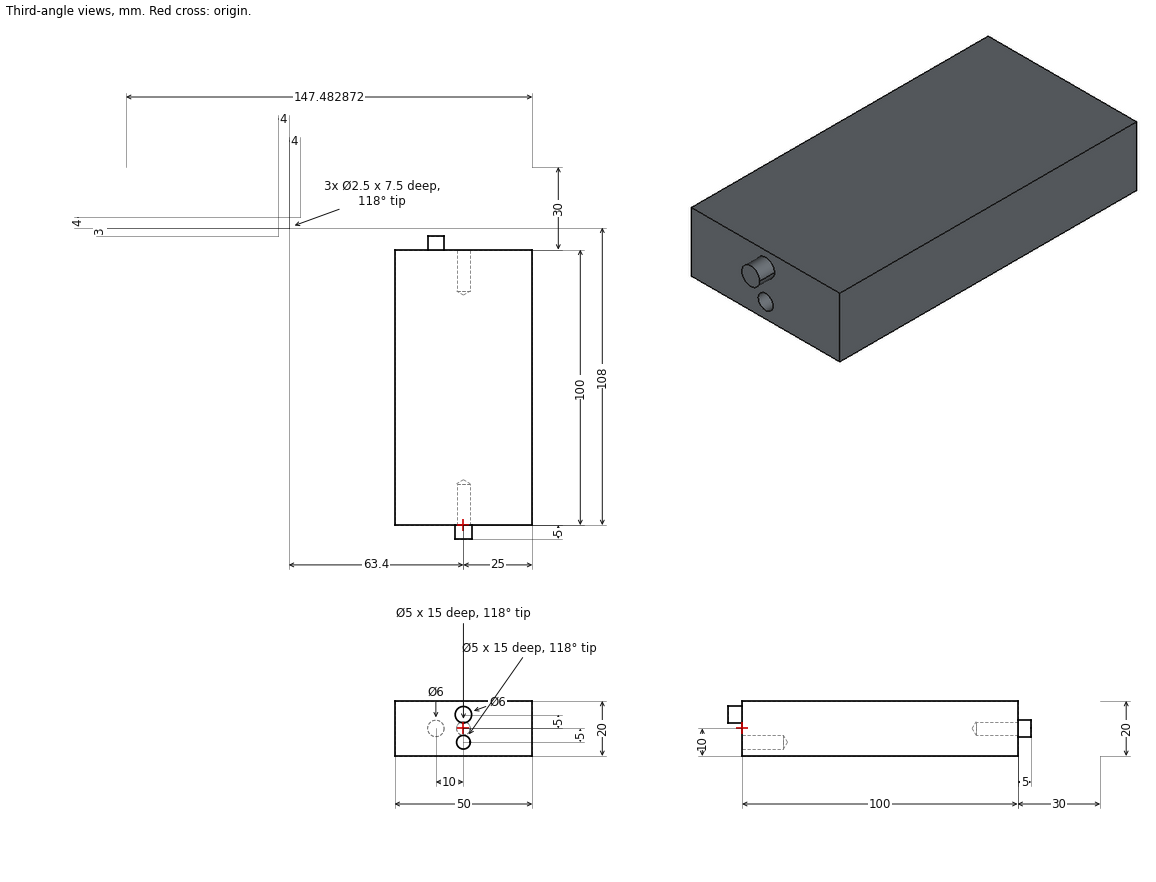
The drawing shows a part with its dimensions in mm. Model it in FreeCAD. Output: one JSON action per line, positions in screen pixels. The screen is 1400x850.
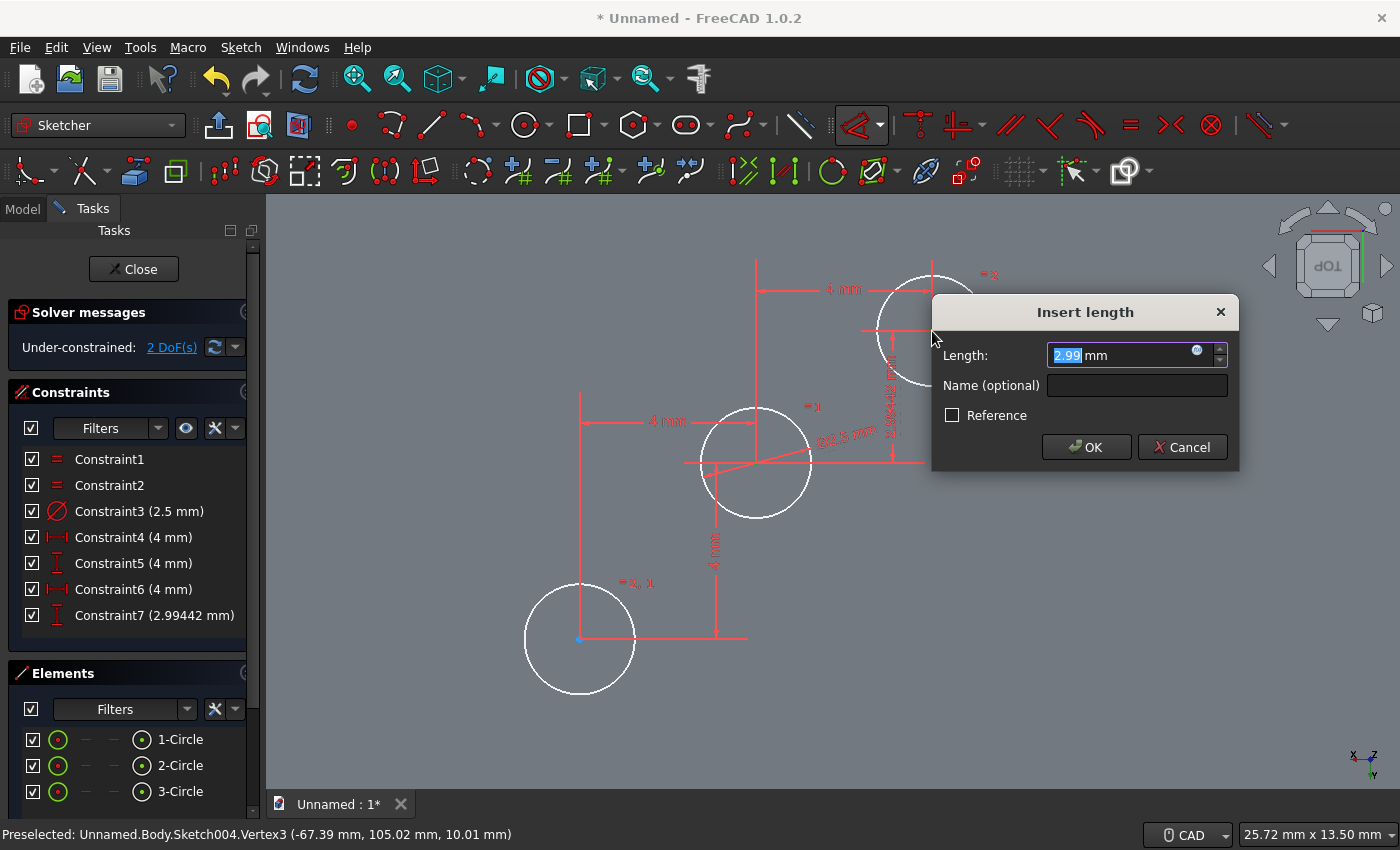
{"action": "type", "text": "3"}
{"action": "key", "text": "Return"}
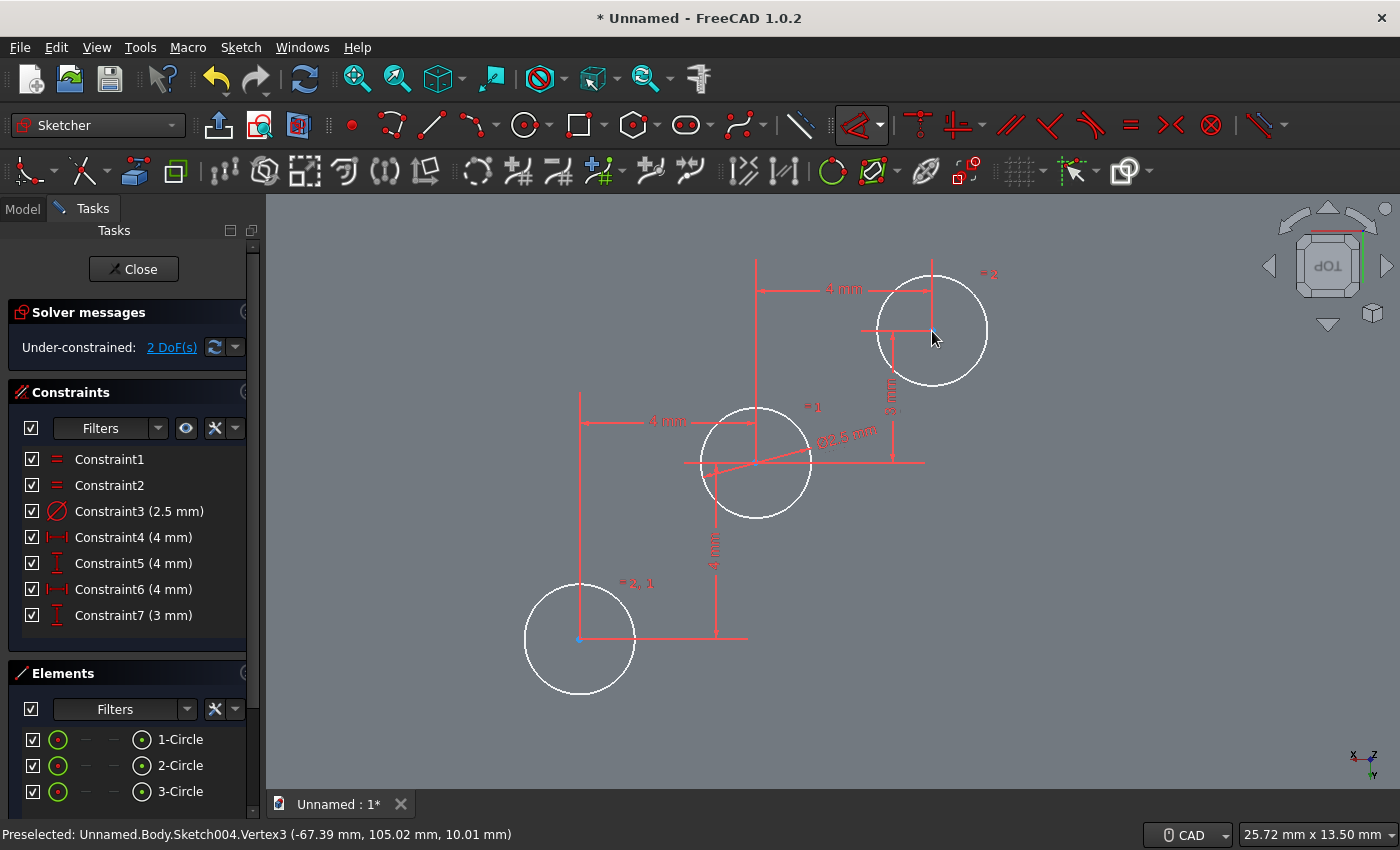
{"action": "left_click", "coordinate": [756, 463]}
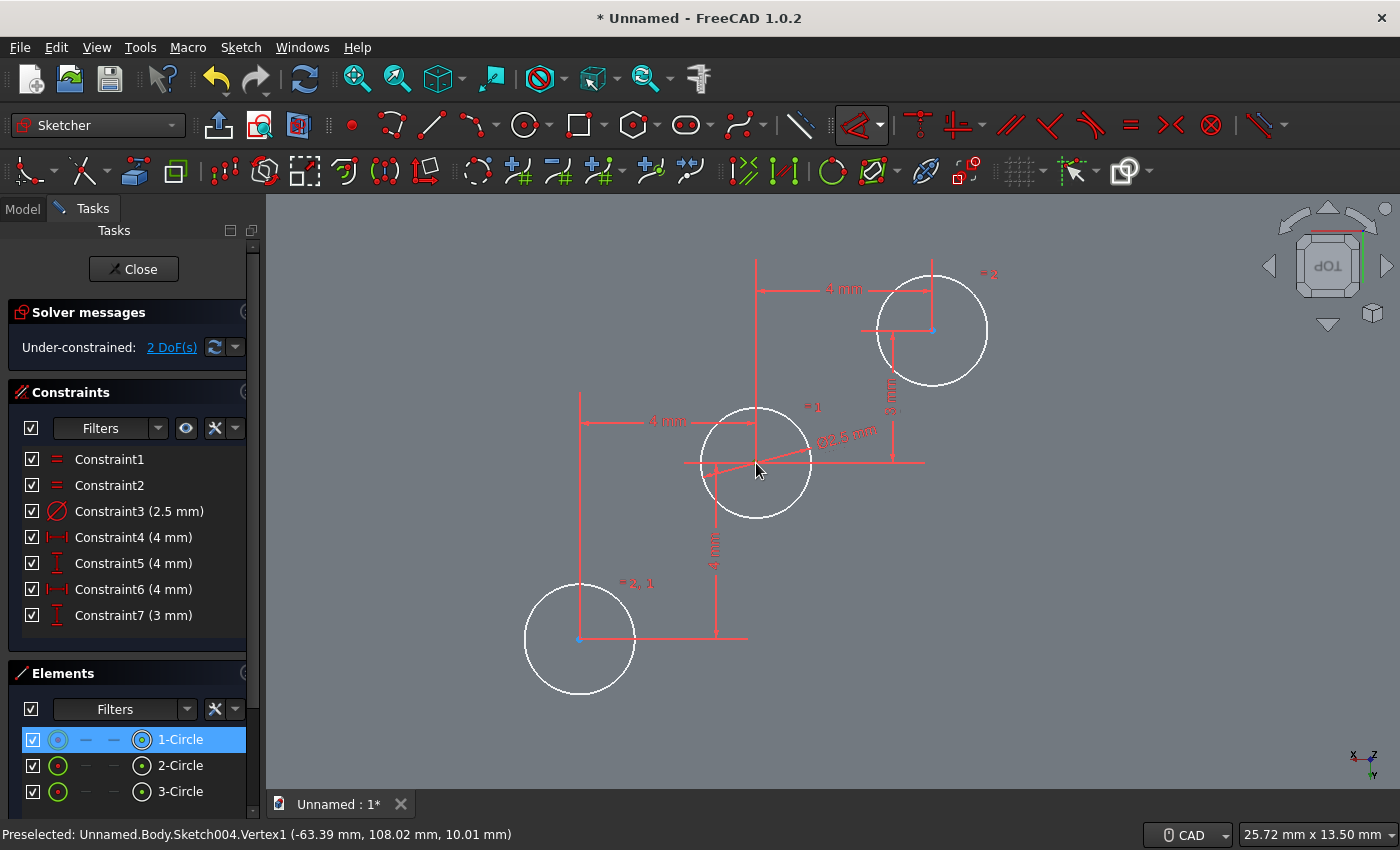
{"action": "key", "text": "i"}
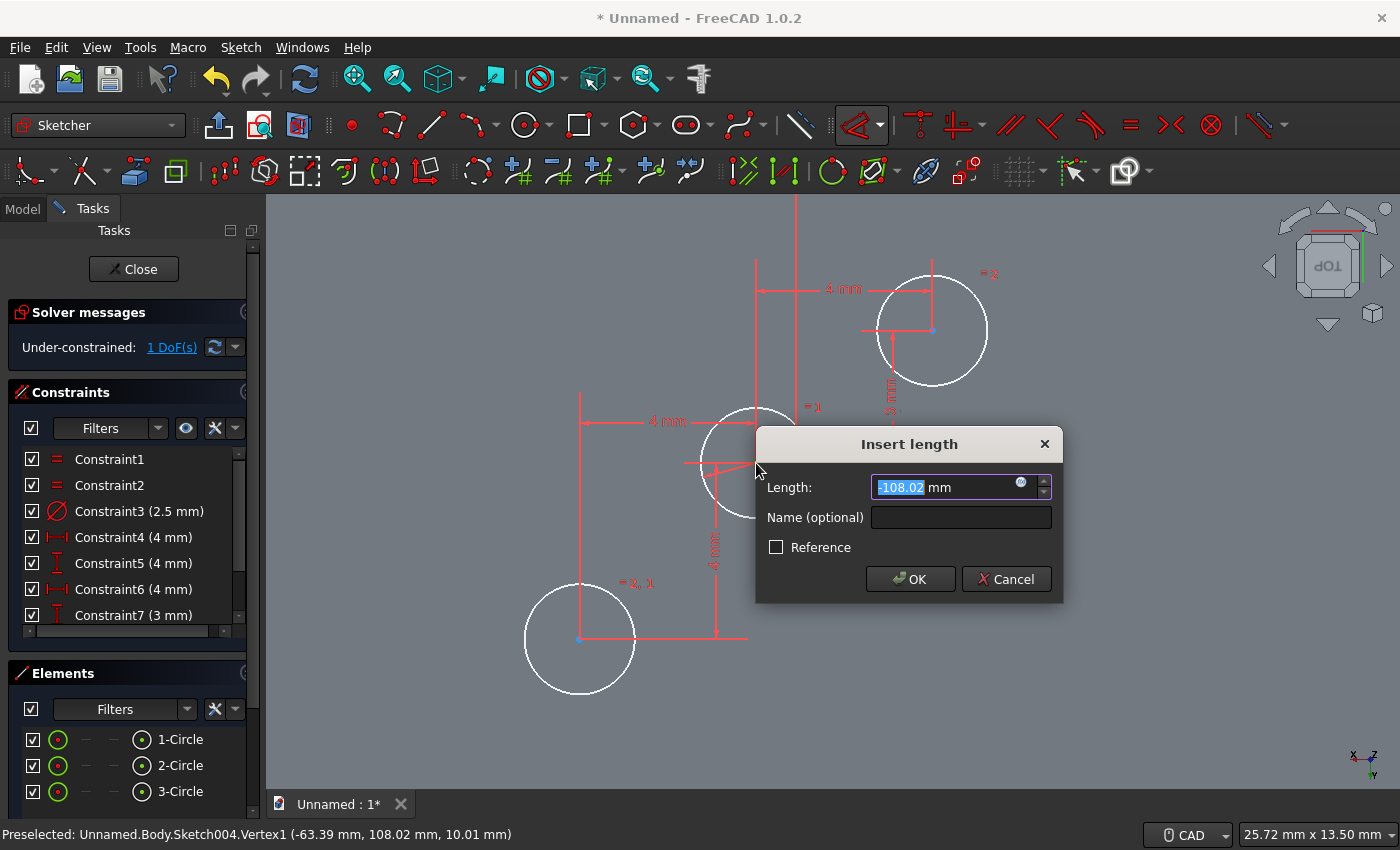
{"action": "type", "text": "-108"}
{"action": "key", "text": "Return"}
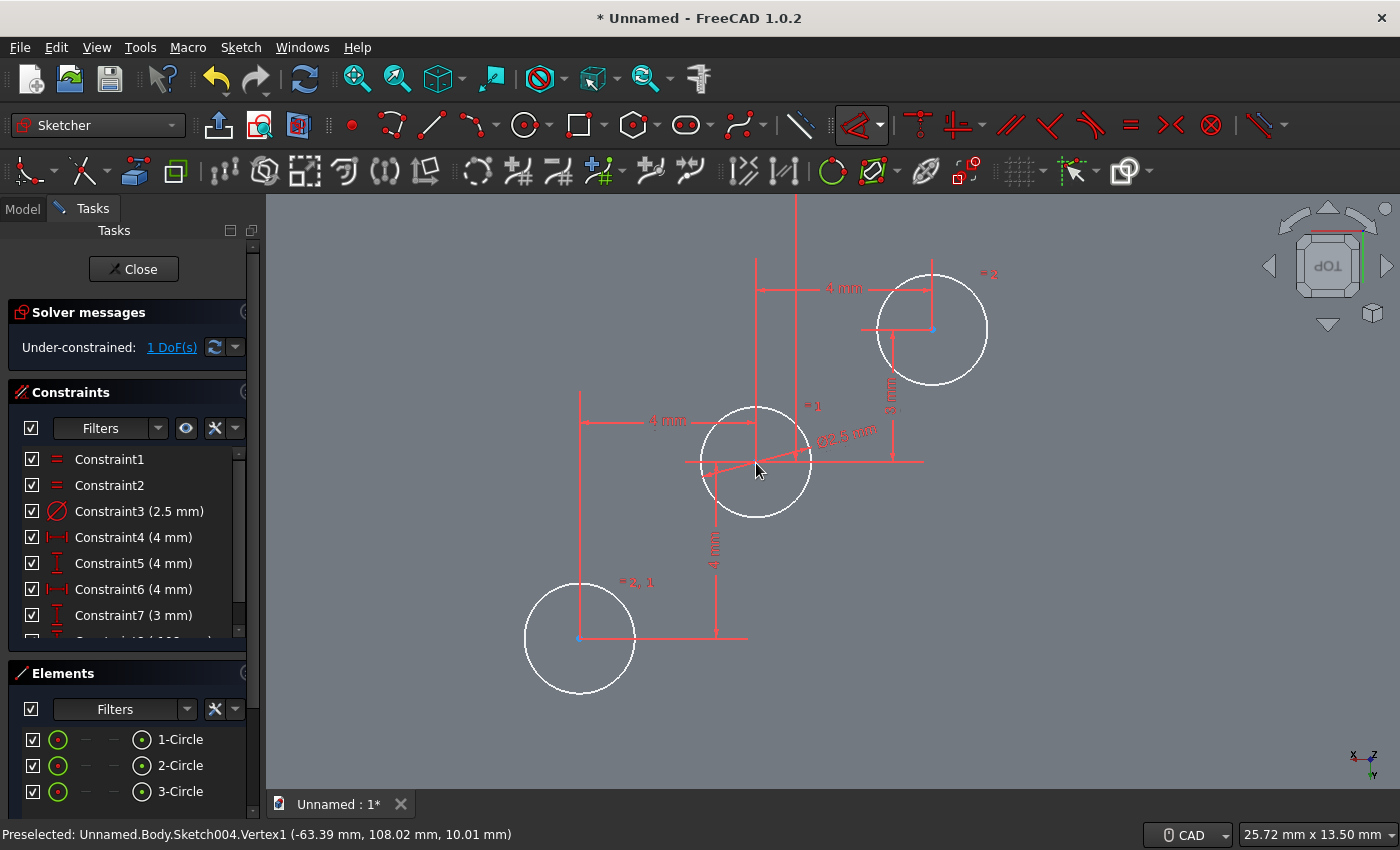
{"action": "left_click", "coordinate": [756, 462]}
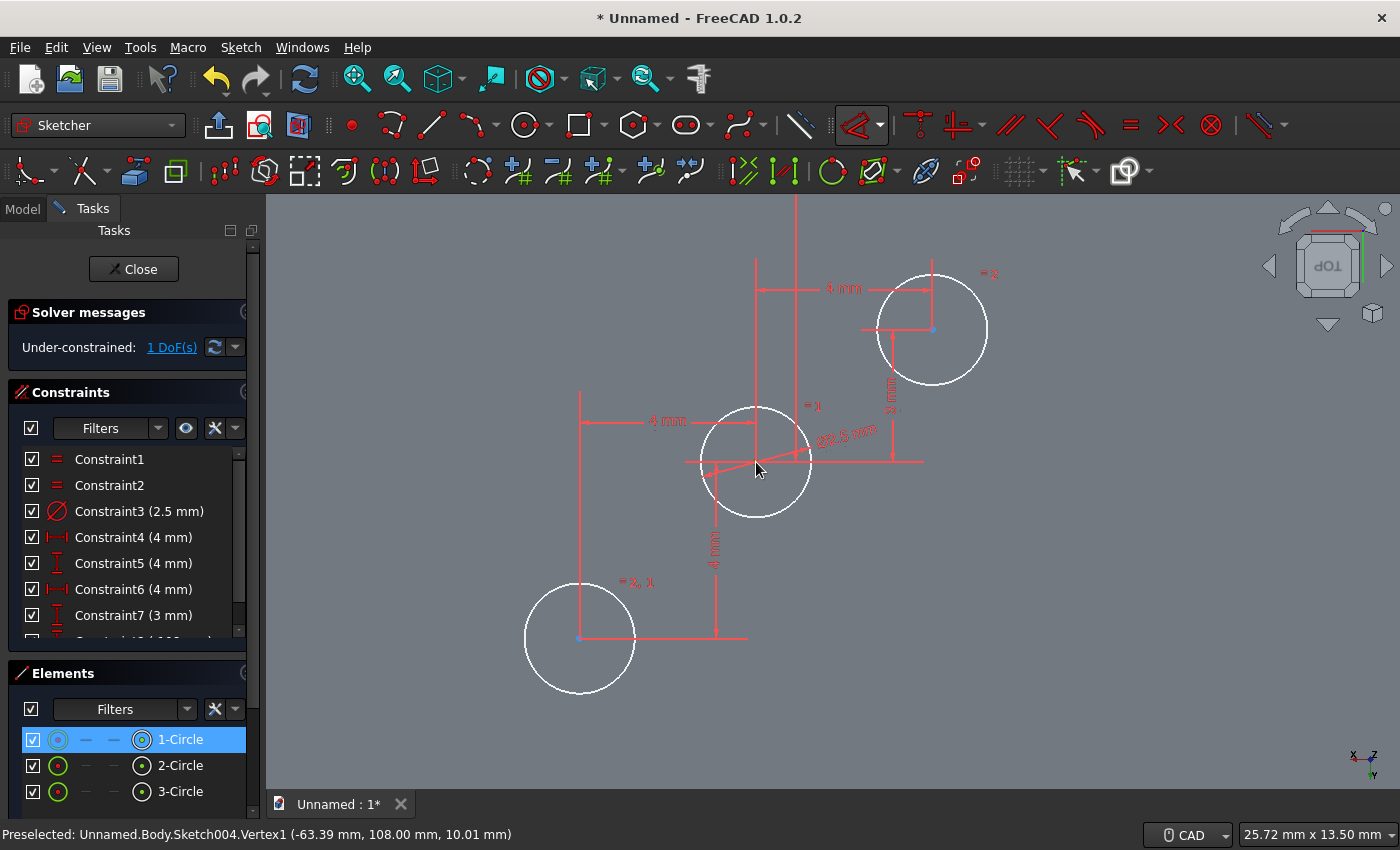
{"action": "key", "text": "l"}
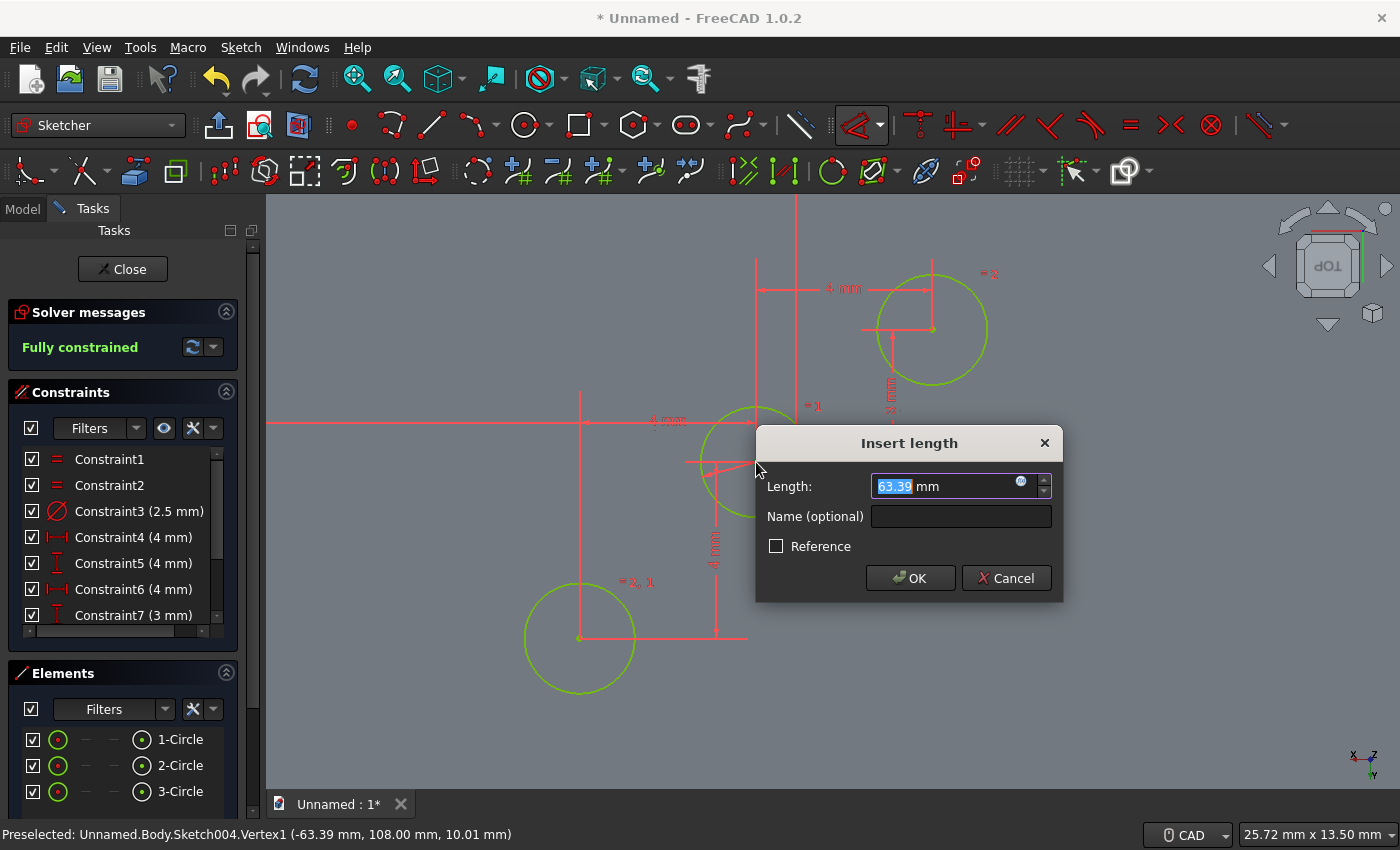
{"action": "type", "text": "63.4"}
{"action": "key", "text": "Return"}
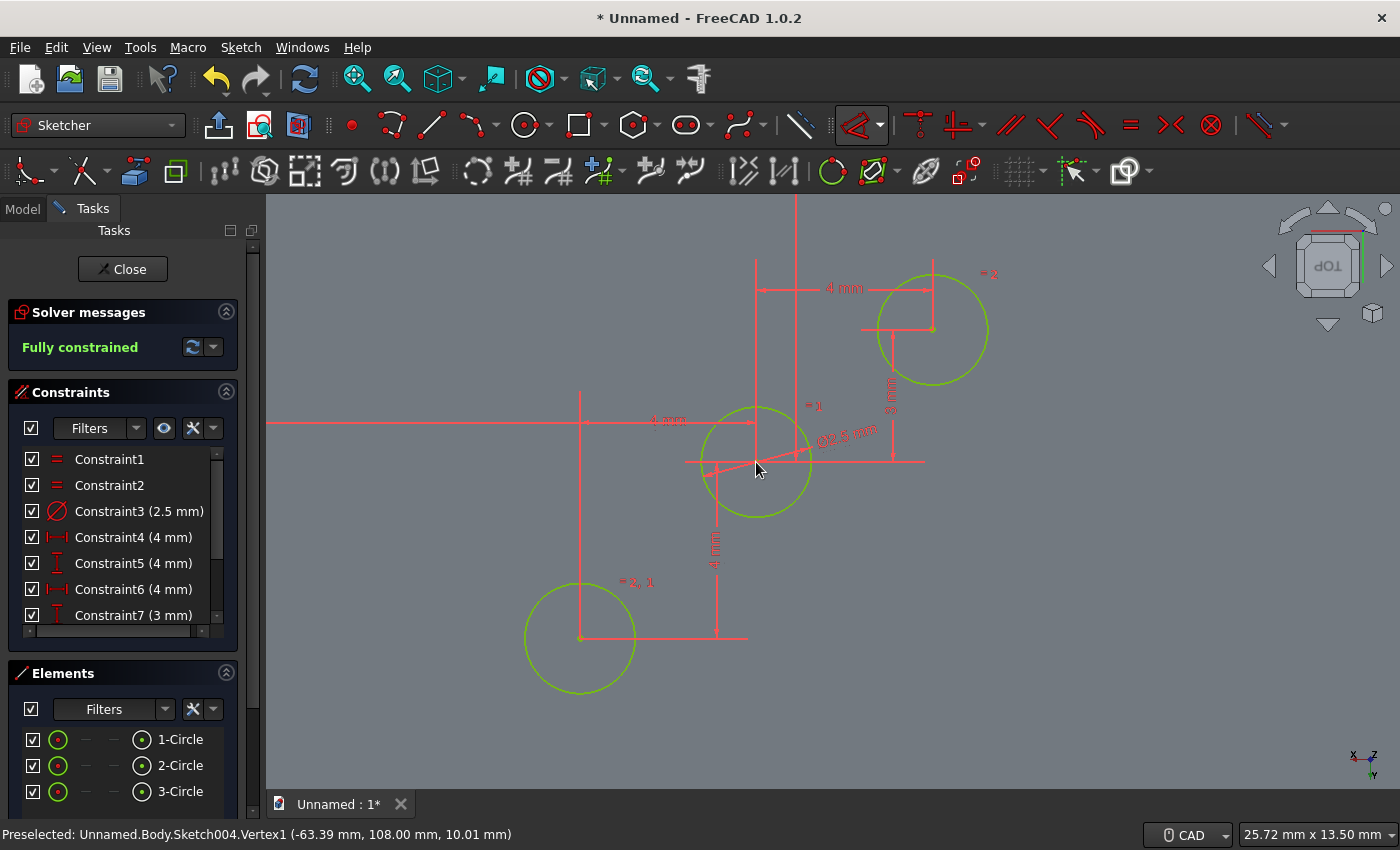
{"action": "left_click", "coordinate": [123, 269]}